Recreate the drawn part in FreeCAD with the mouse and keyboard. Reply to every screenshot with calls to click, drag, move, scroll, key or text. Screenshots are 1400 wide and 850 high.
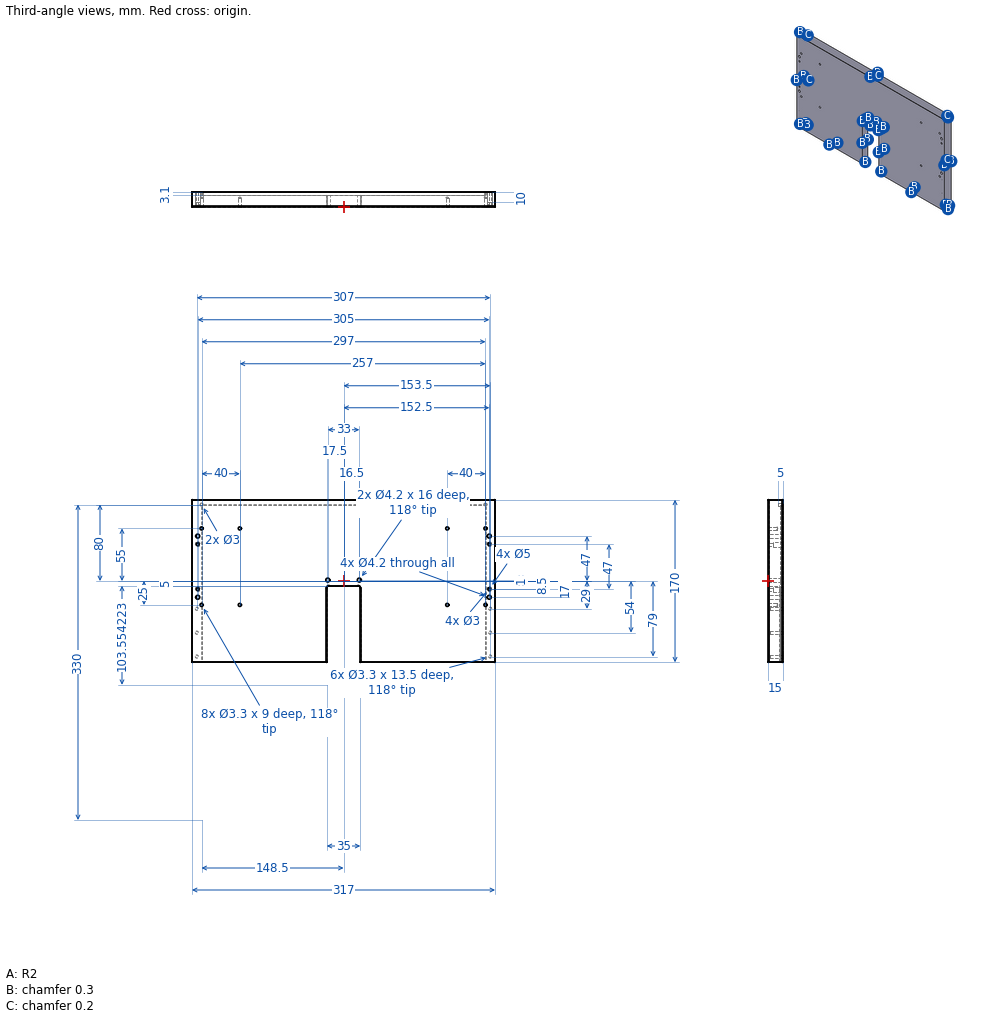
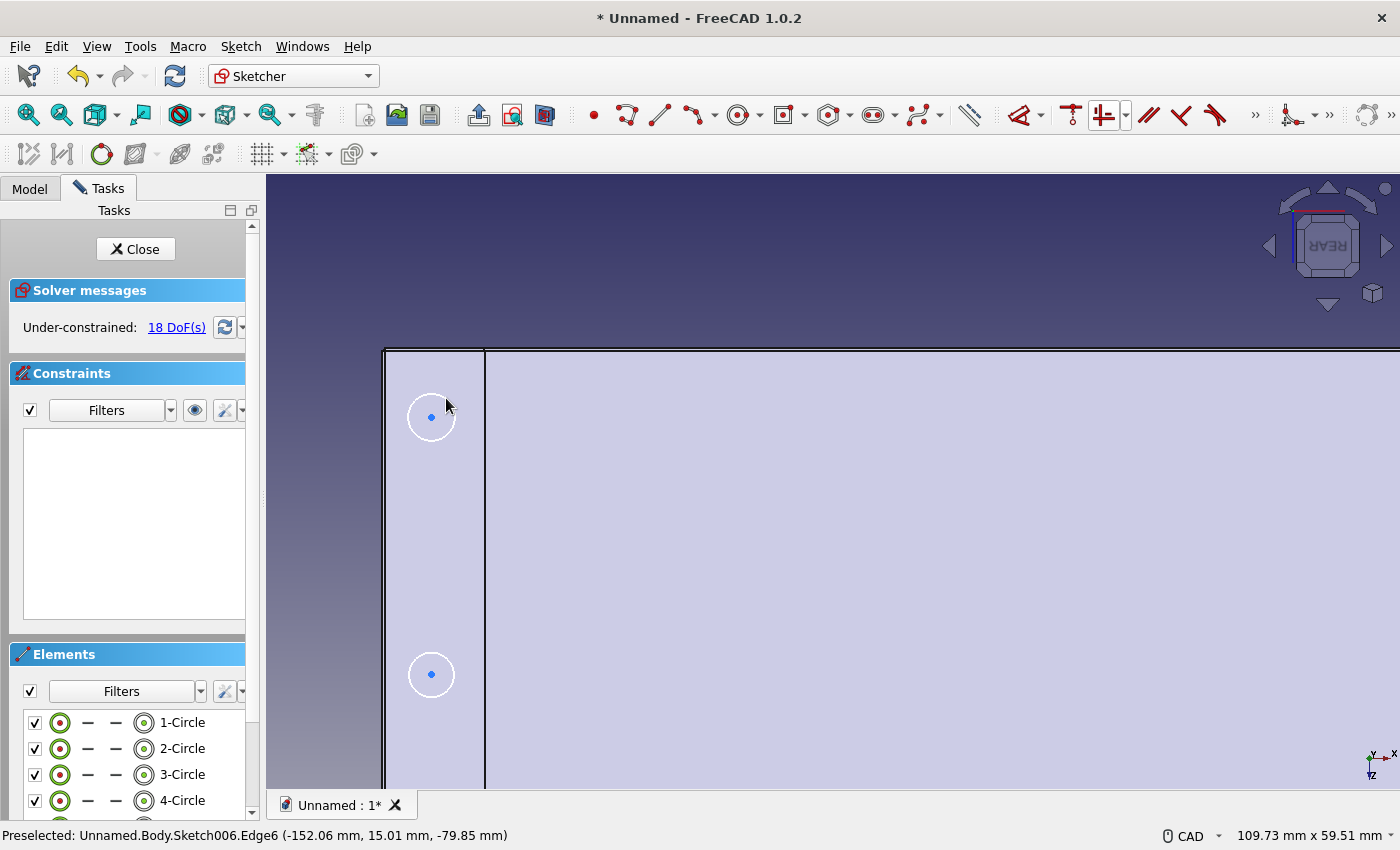
scroll(447, 398, down, 8)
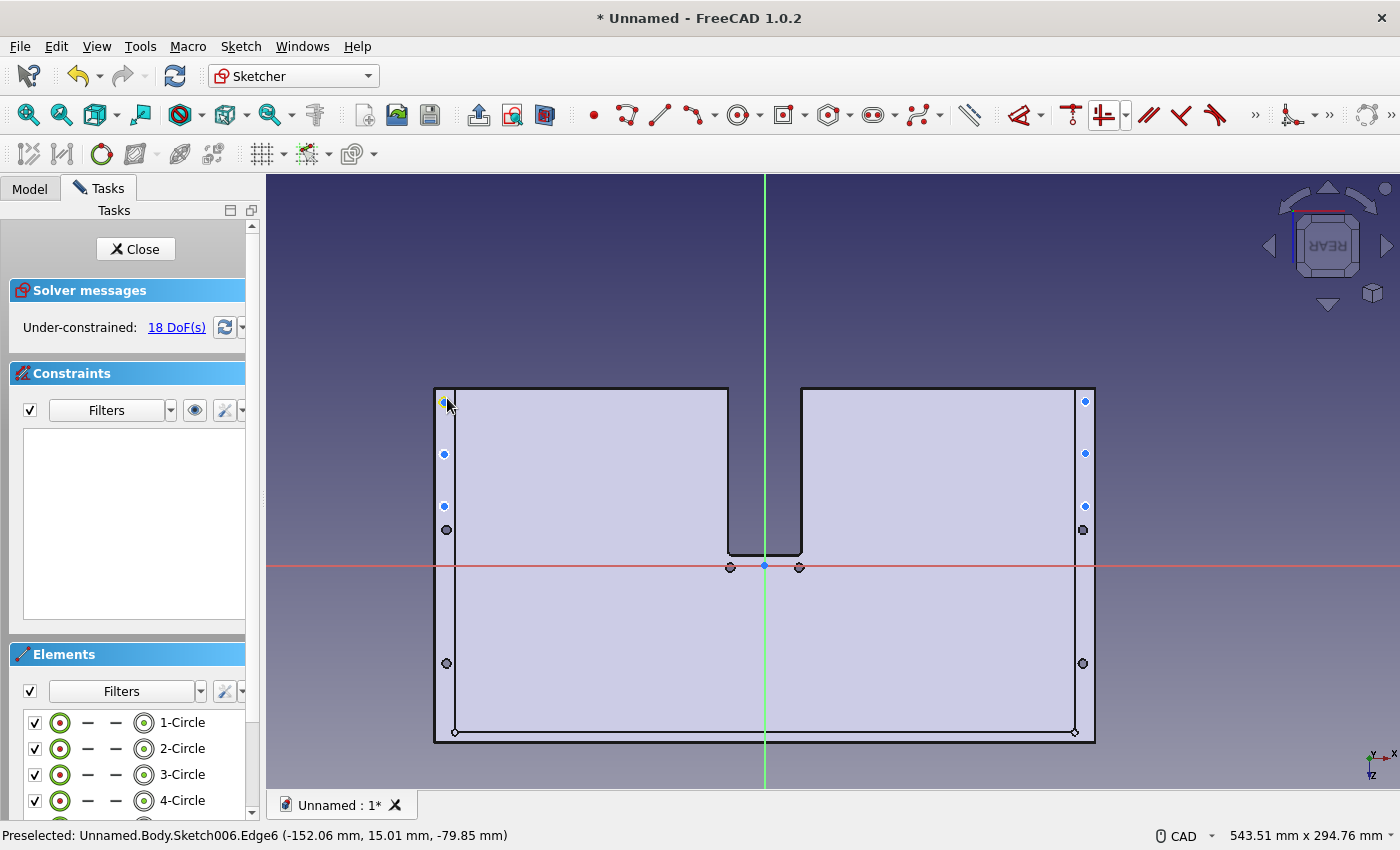
scroll(1088, 399, up, 7)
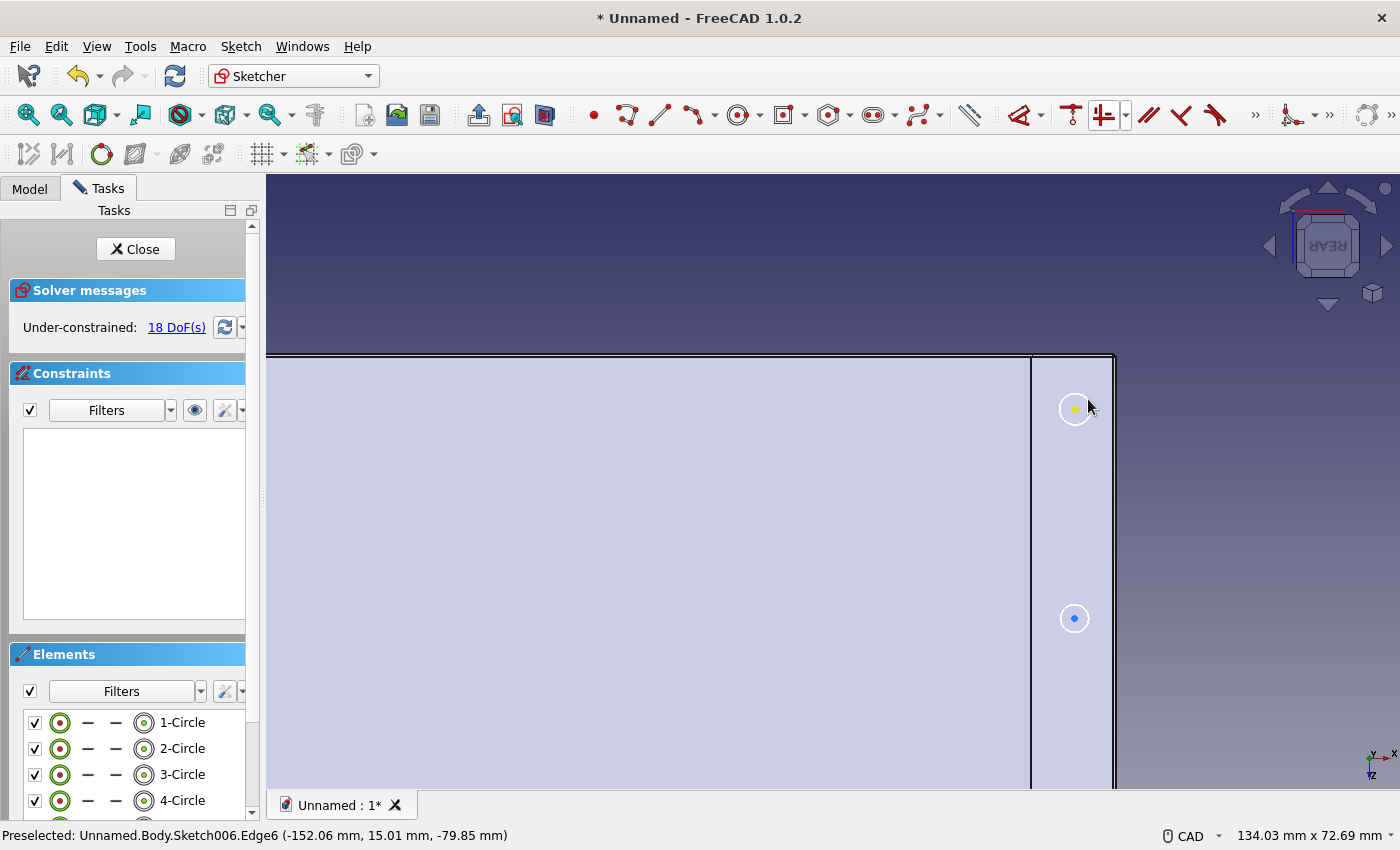
click(1086, 398)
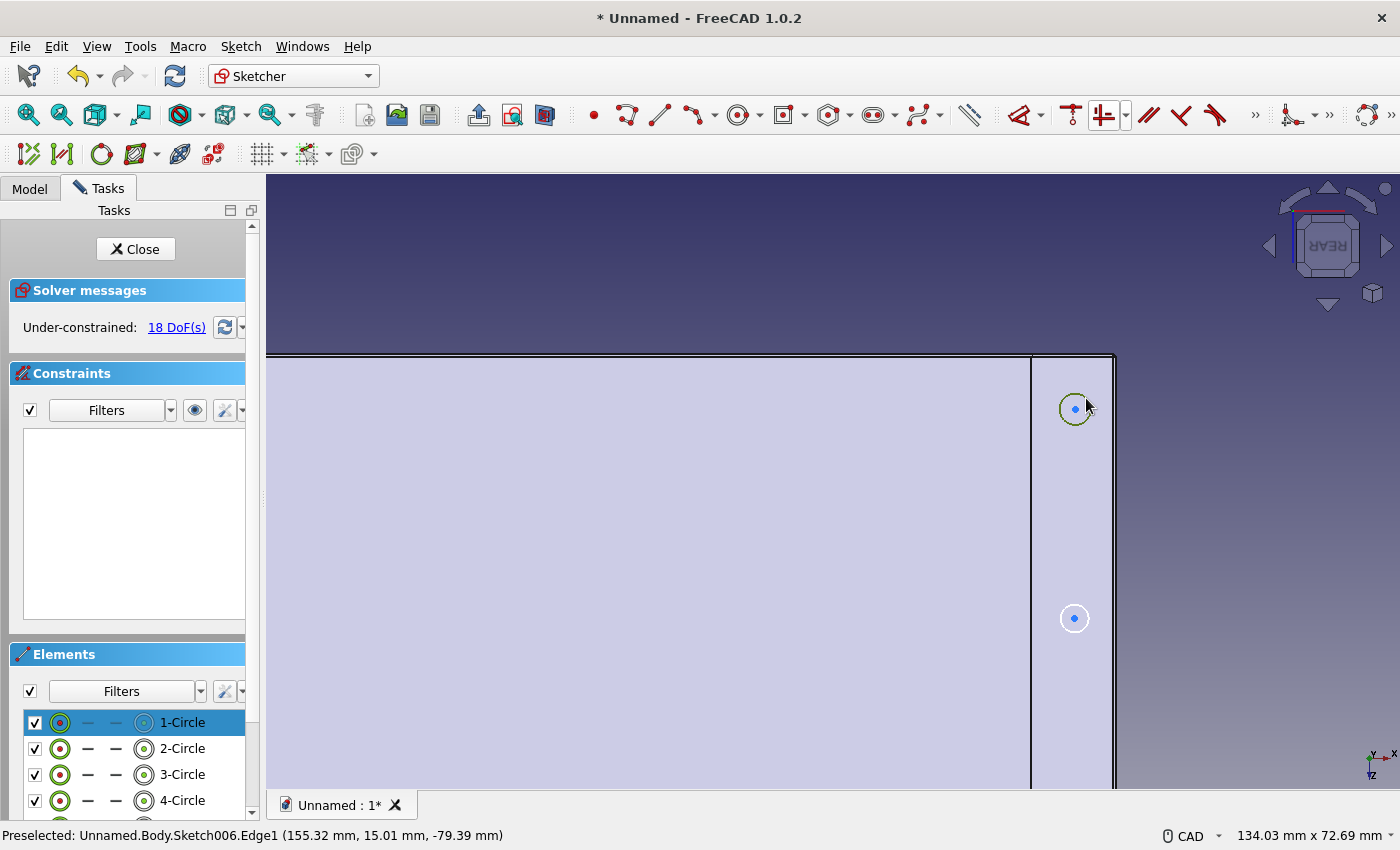
click(1084, 609)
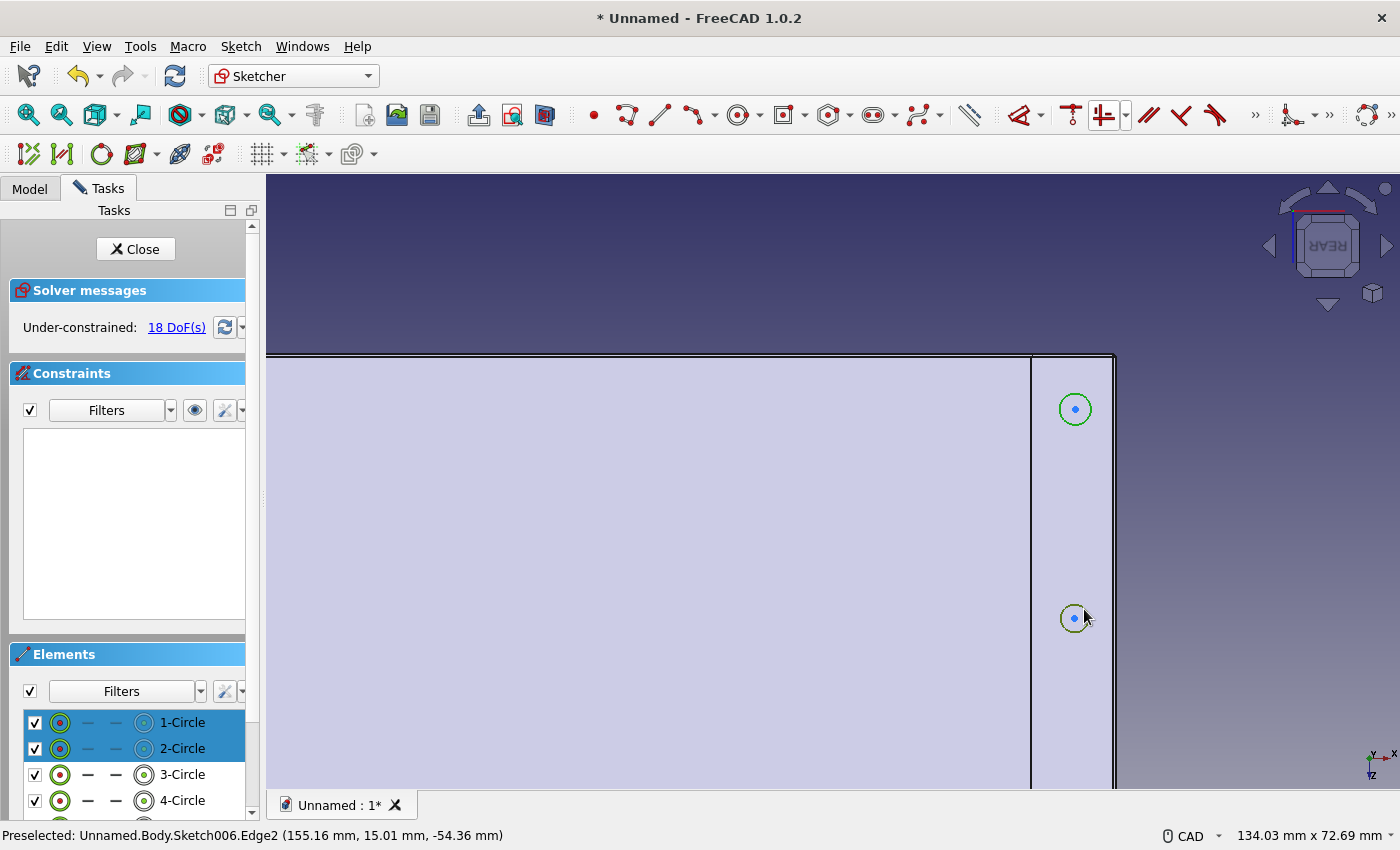
scroll(1088, 399, down, 7)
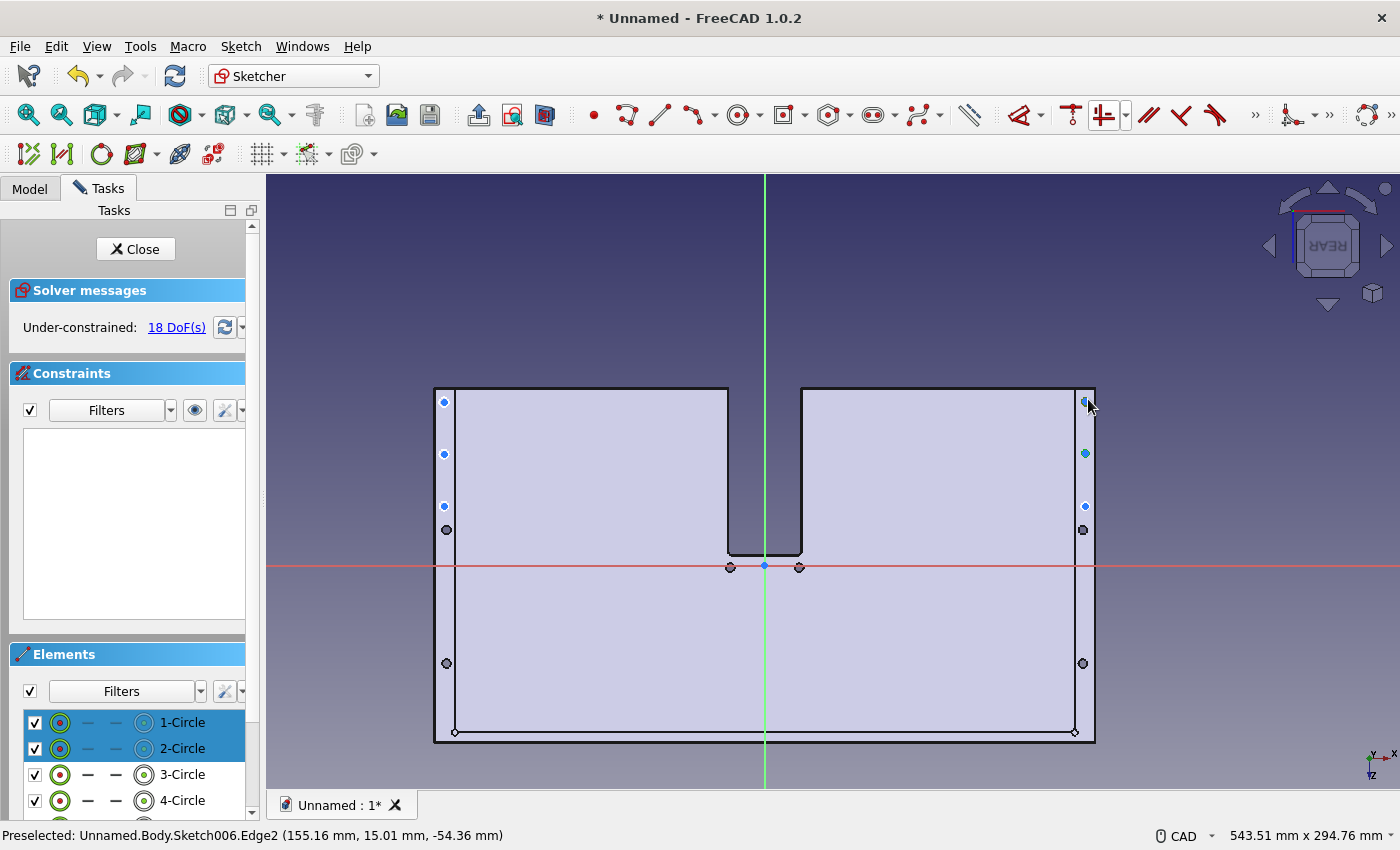
scroll(1088, 503, up, 7)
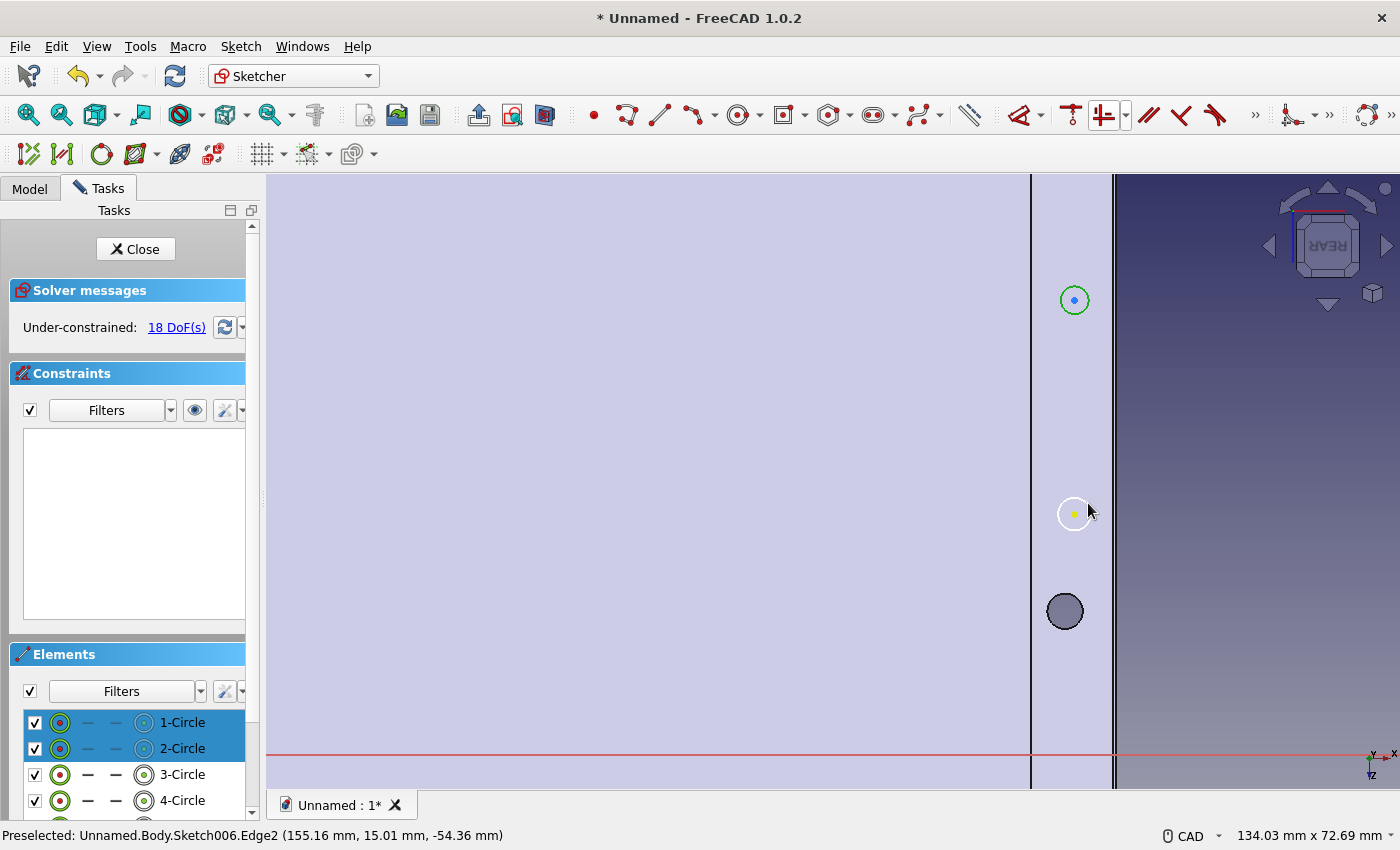
click(1086, 503)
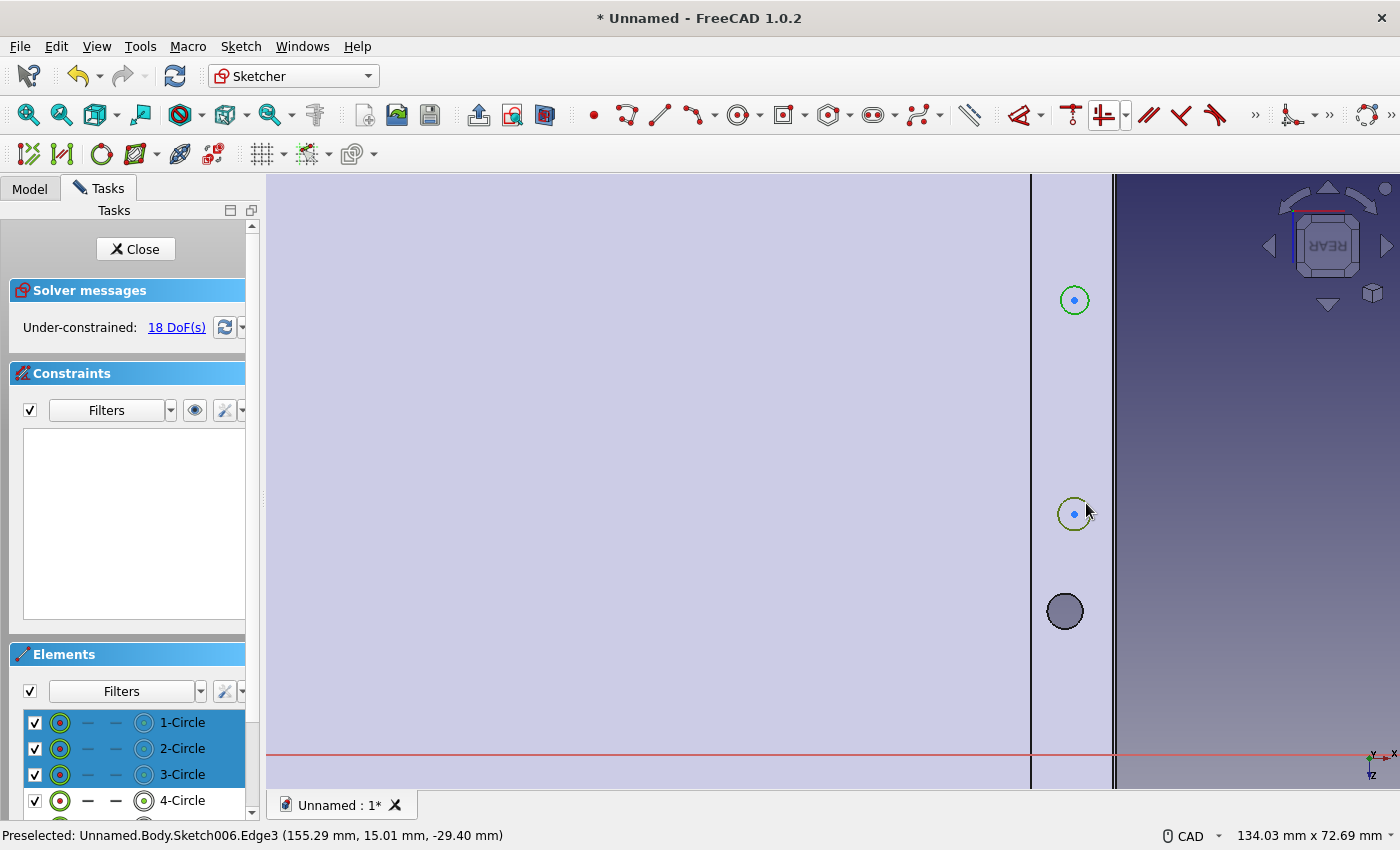
scroll(1088, 504, down, 7)